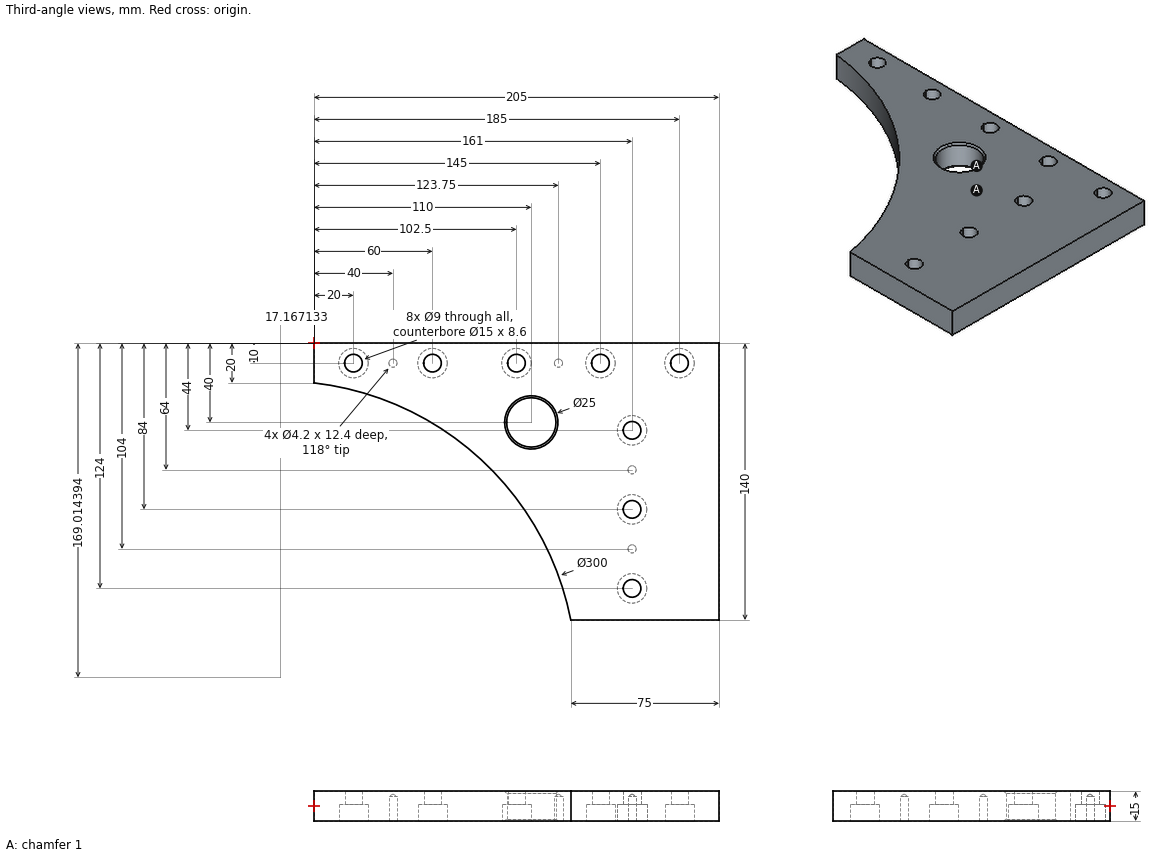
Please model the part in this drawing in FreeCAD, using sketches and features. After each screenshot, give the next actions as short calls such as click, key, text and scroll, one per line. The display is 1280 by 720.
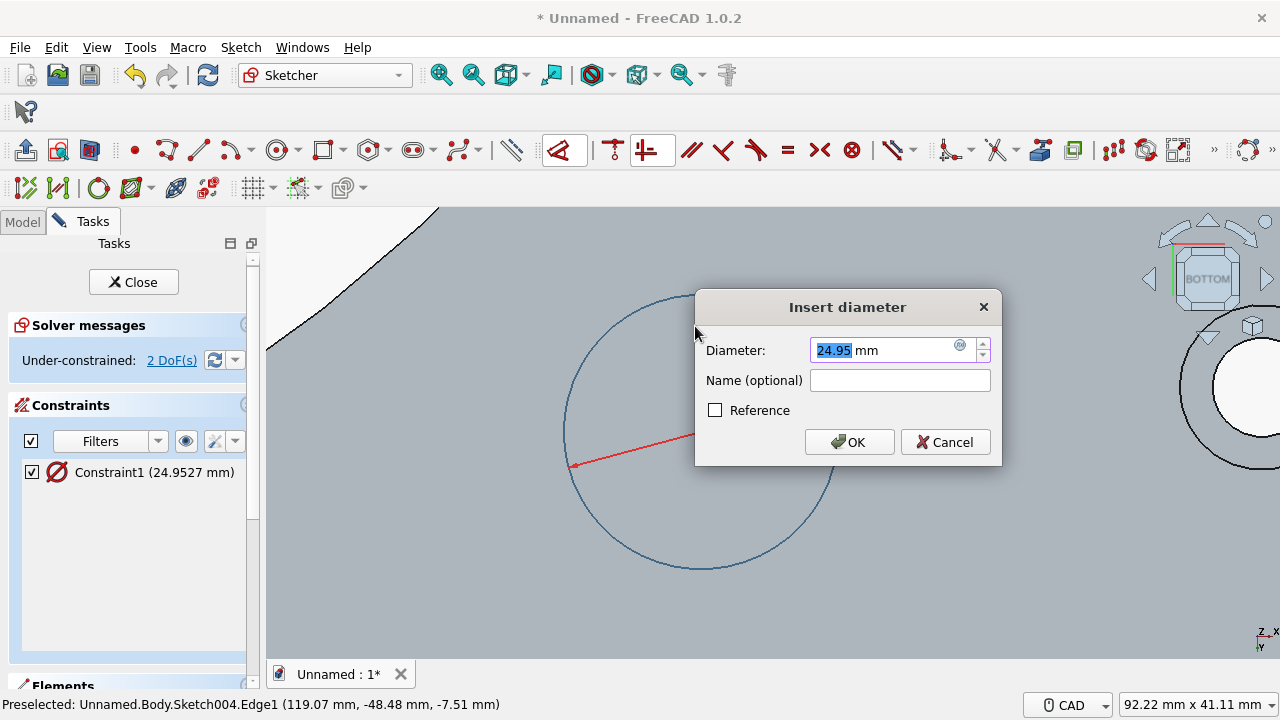
text(25)
key(Return)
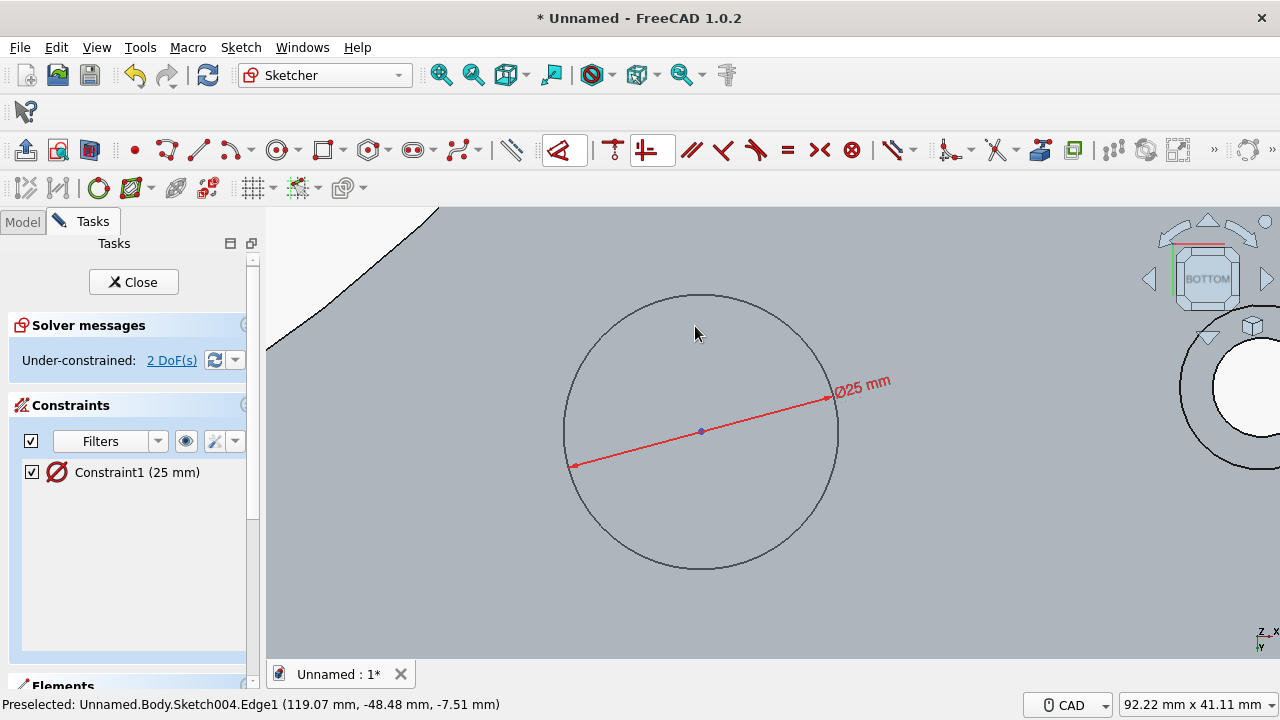
click(701, 432)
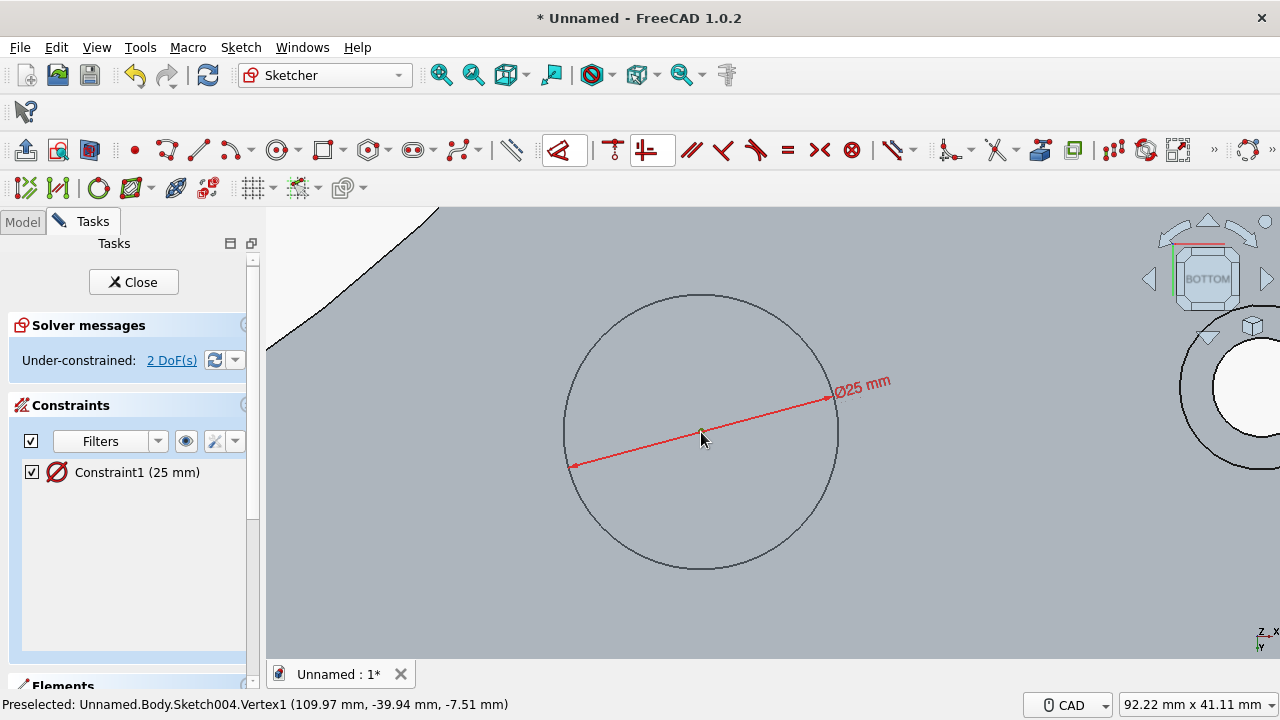
key(i)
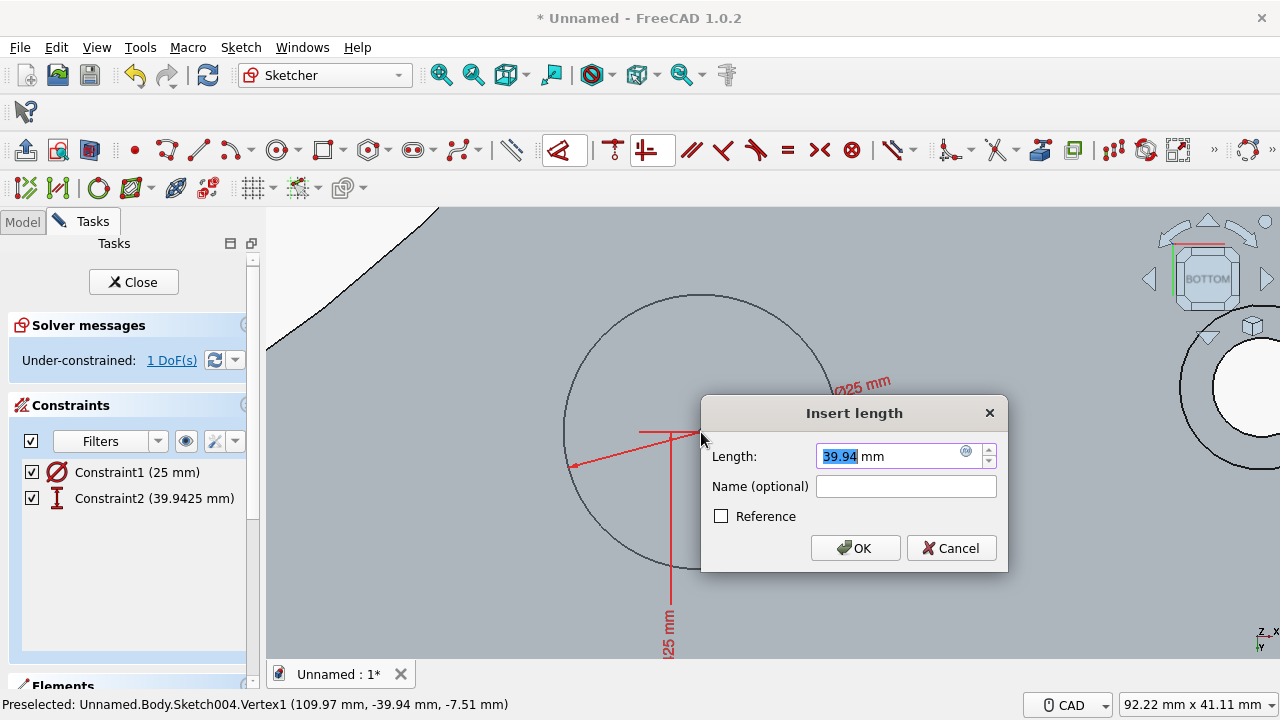
text(40)
key(Return)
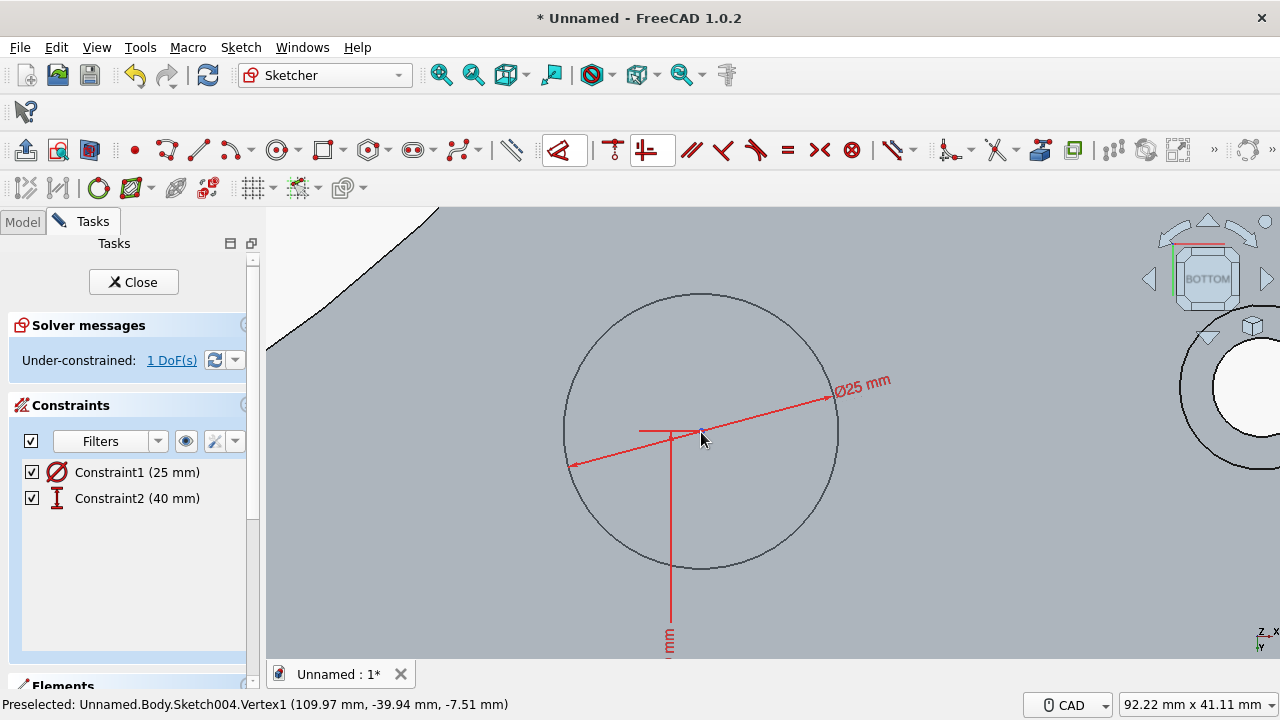
click(701, 431)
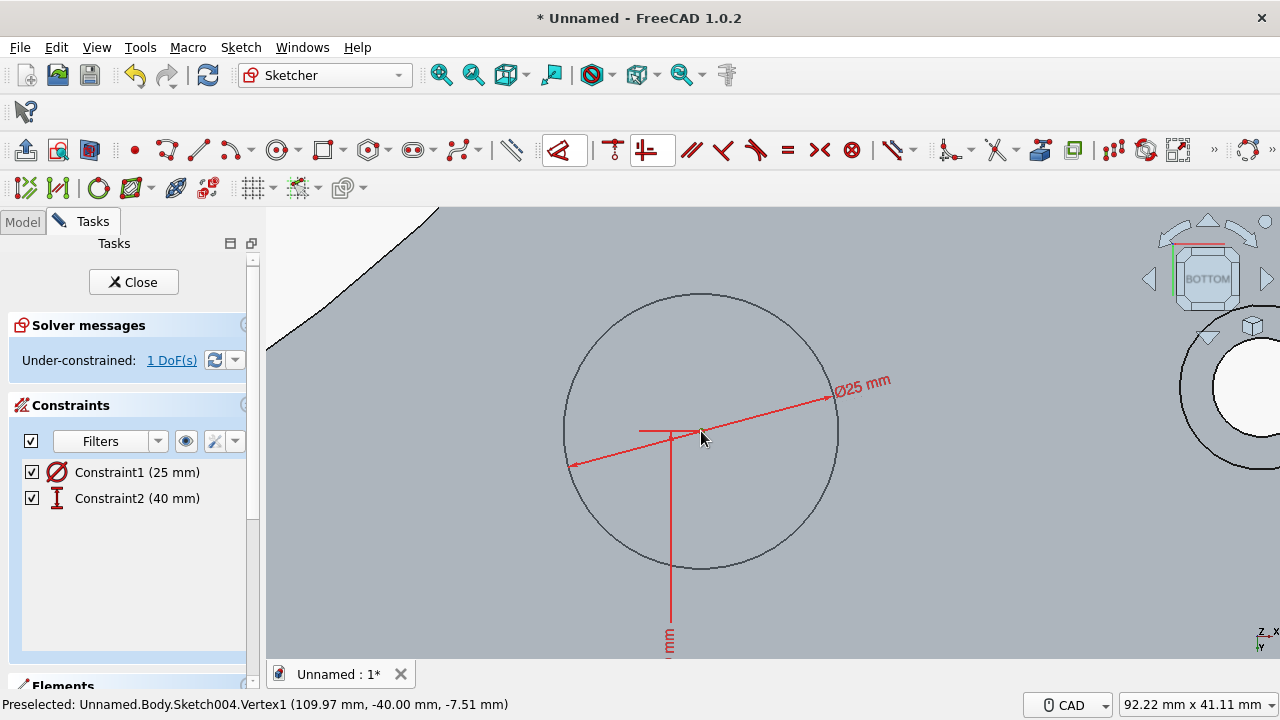
key(l)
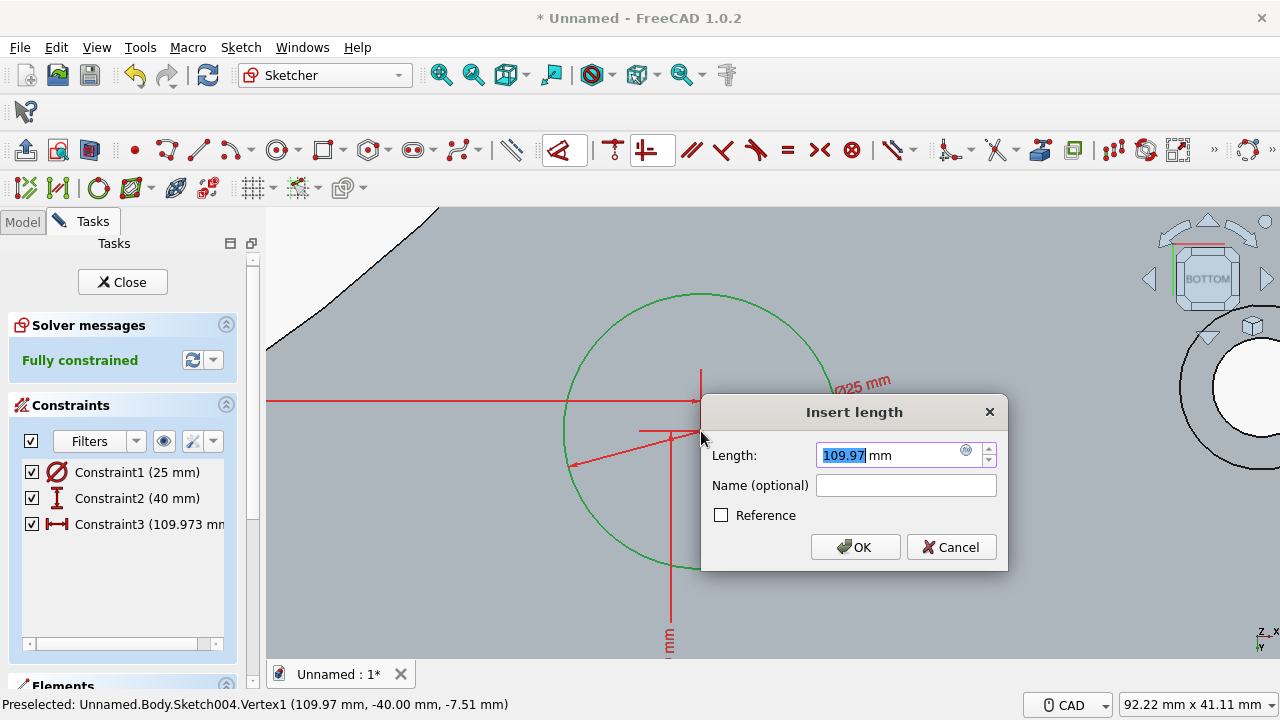
text(110)
key(Return)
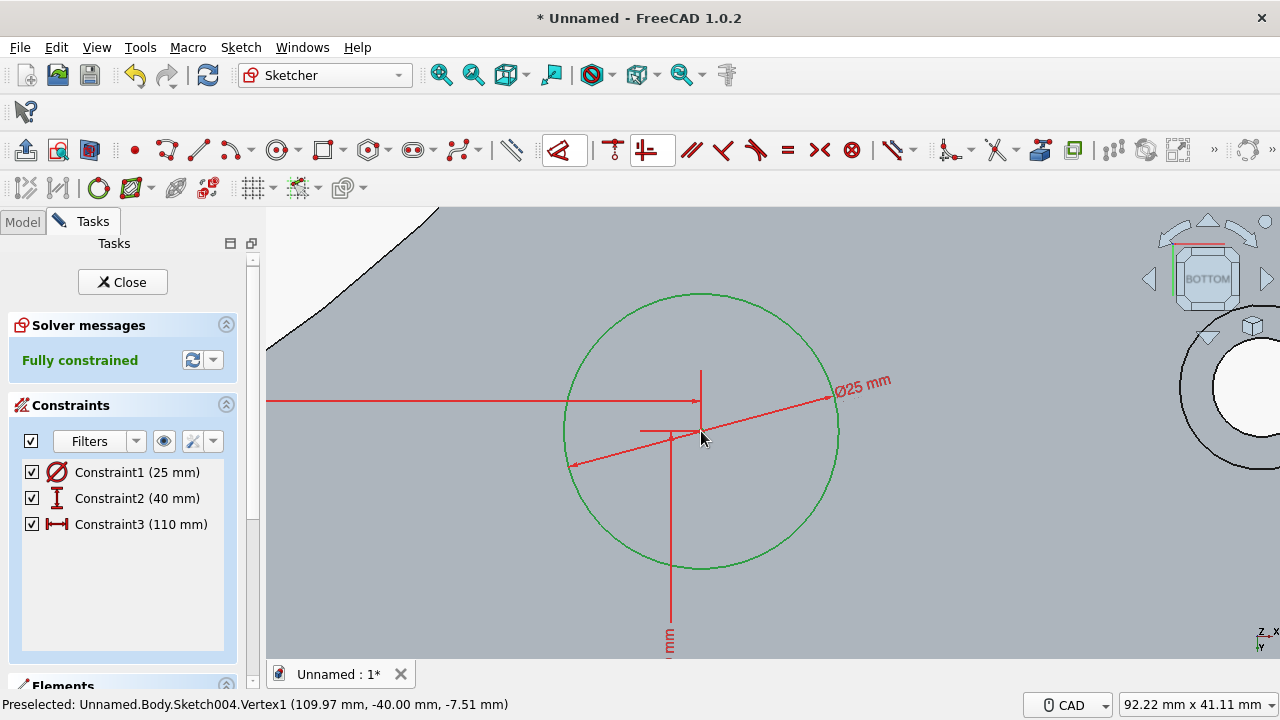
click(123, 282)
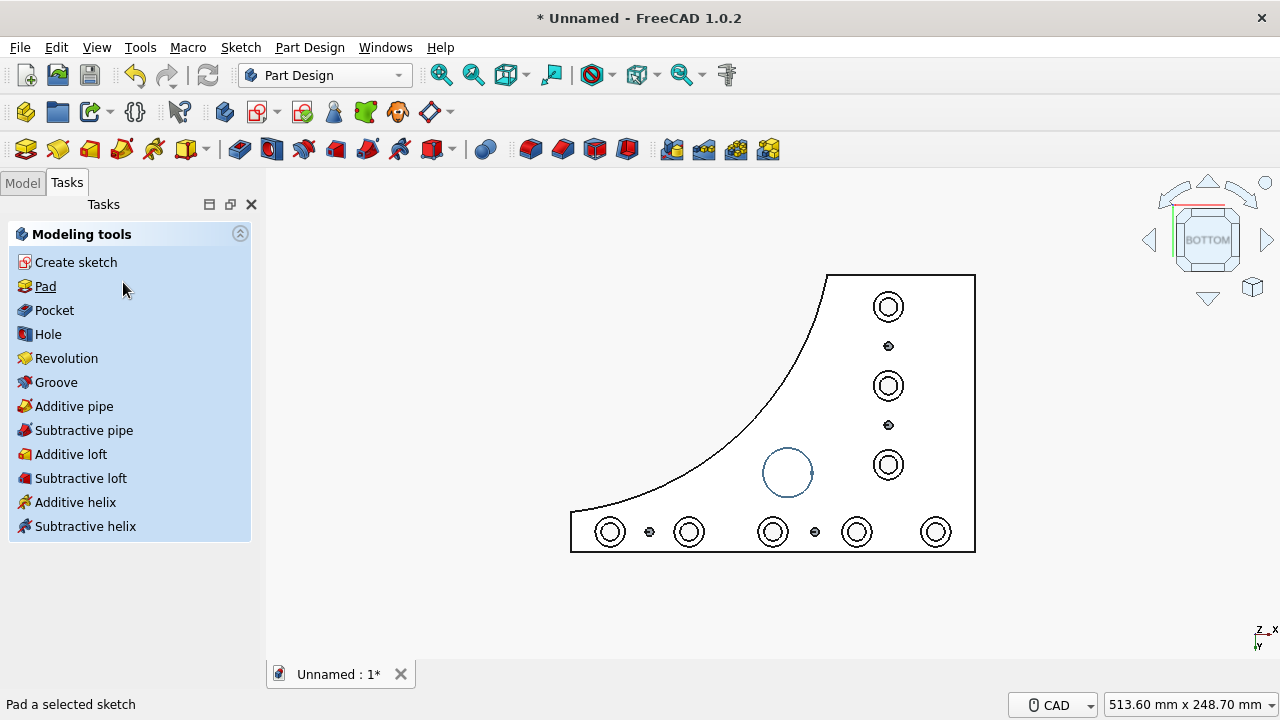
click(240, 150)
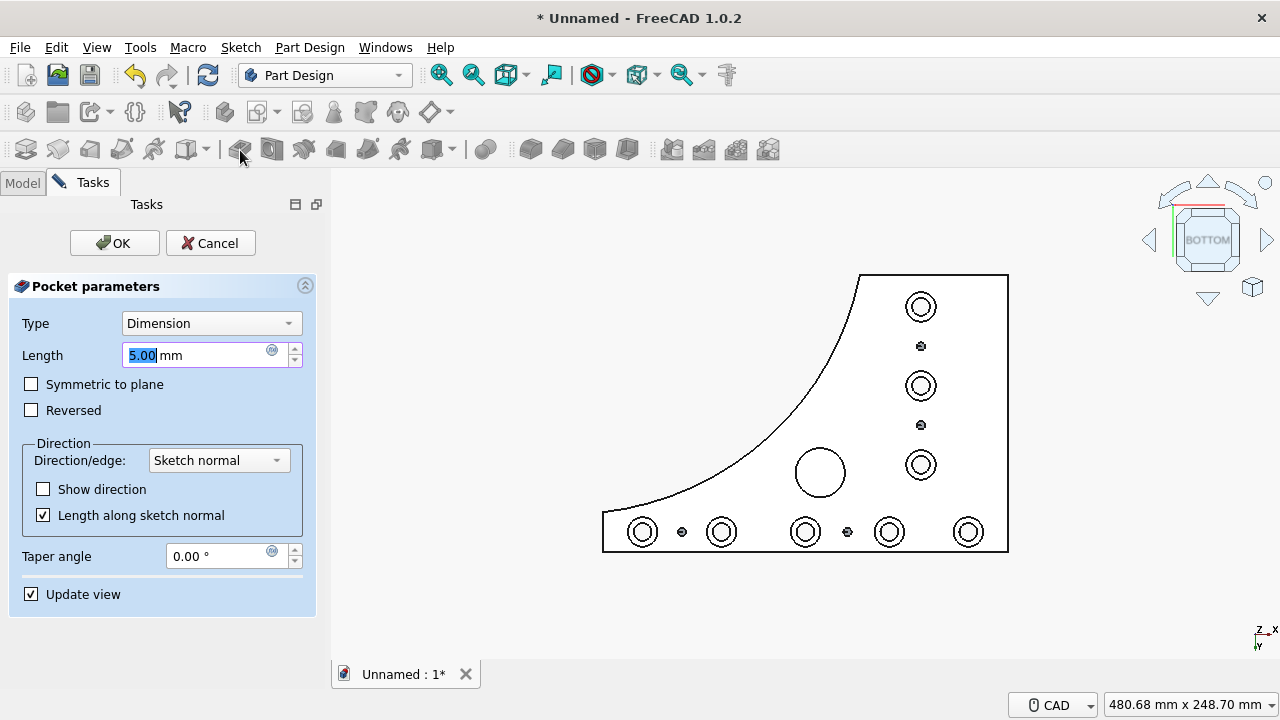
click(212, 324)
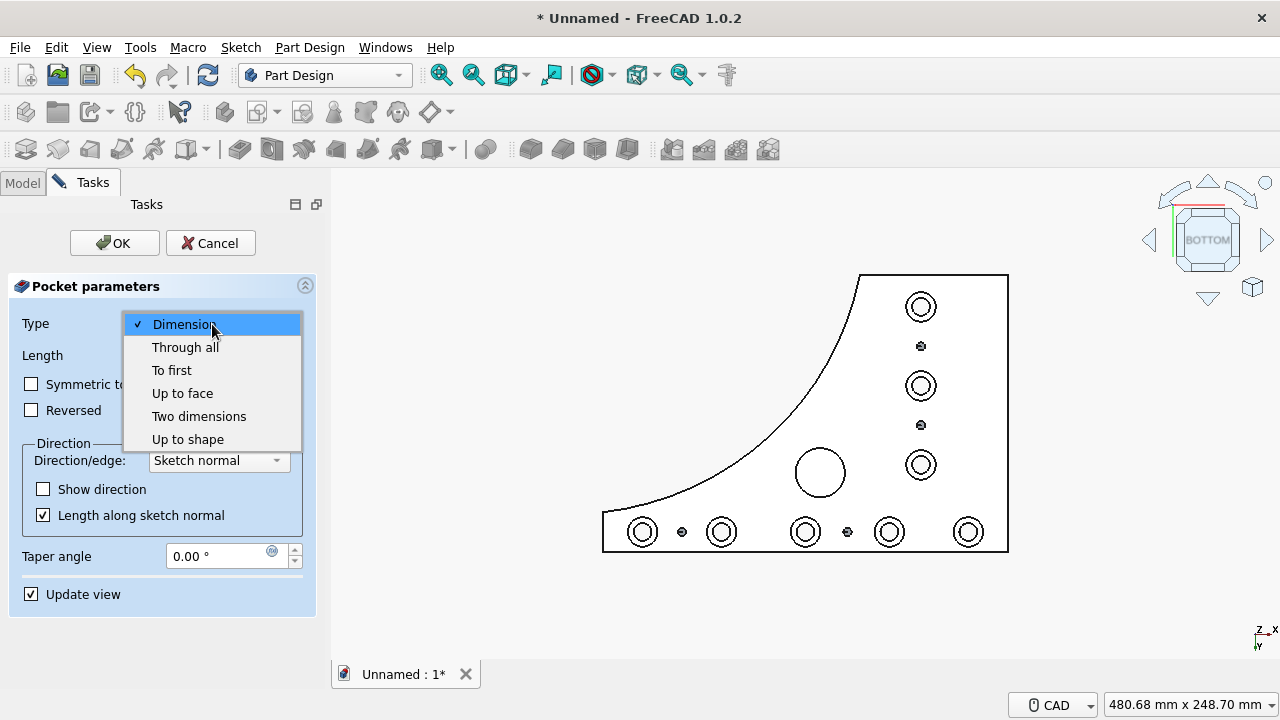
click(212, 348)